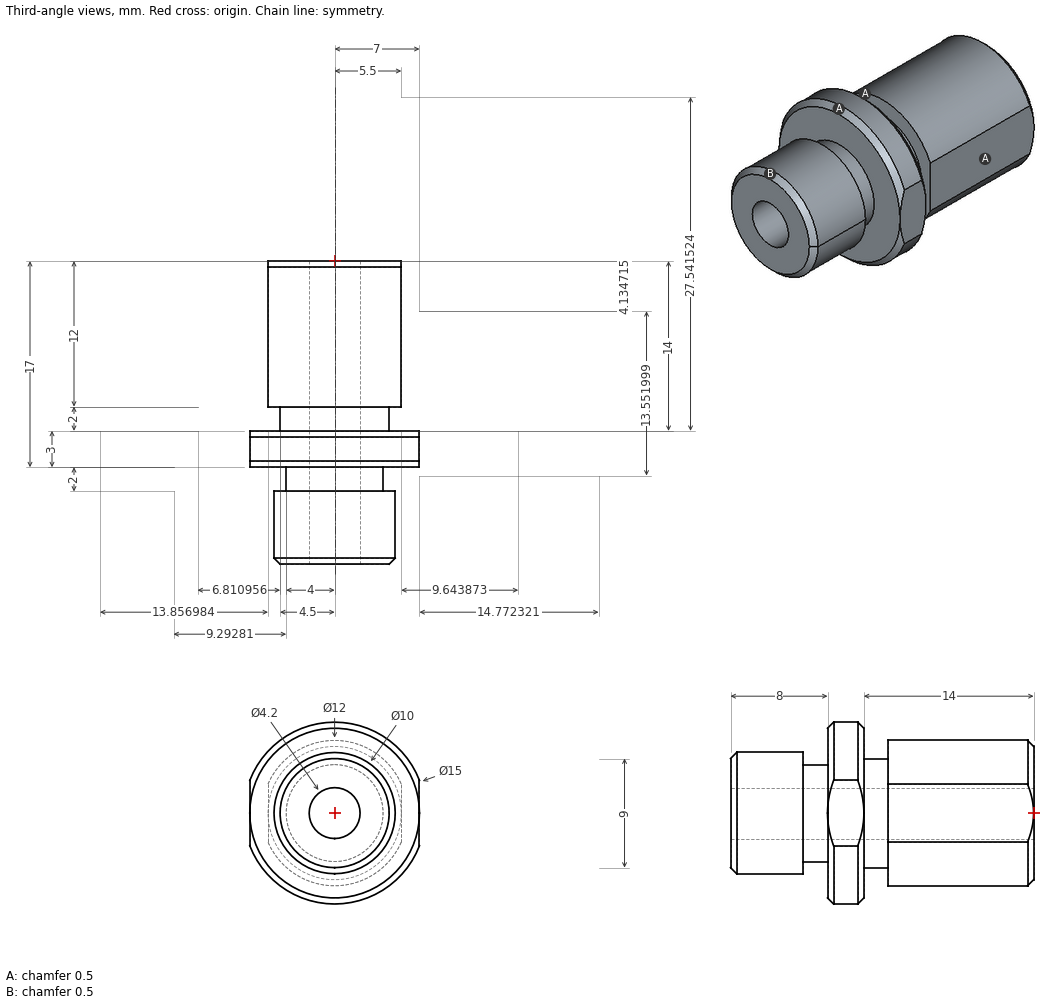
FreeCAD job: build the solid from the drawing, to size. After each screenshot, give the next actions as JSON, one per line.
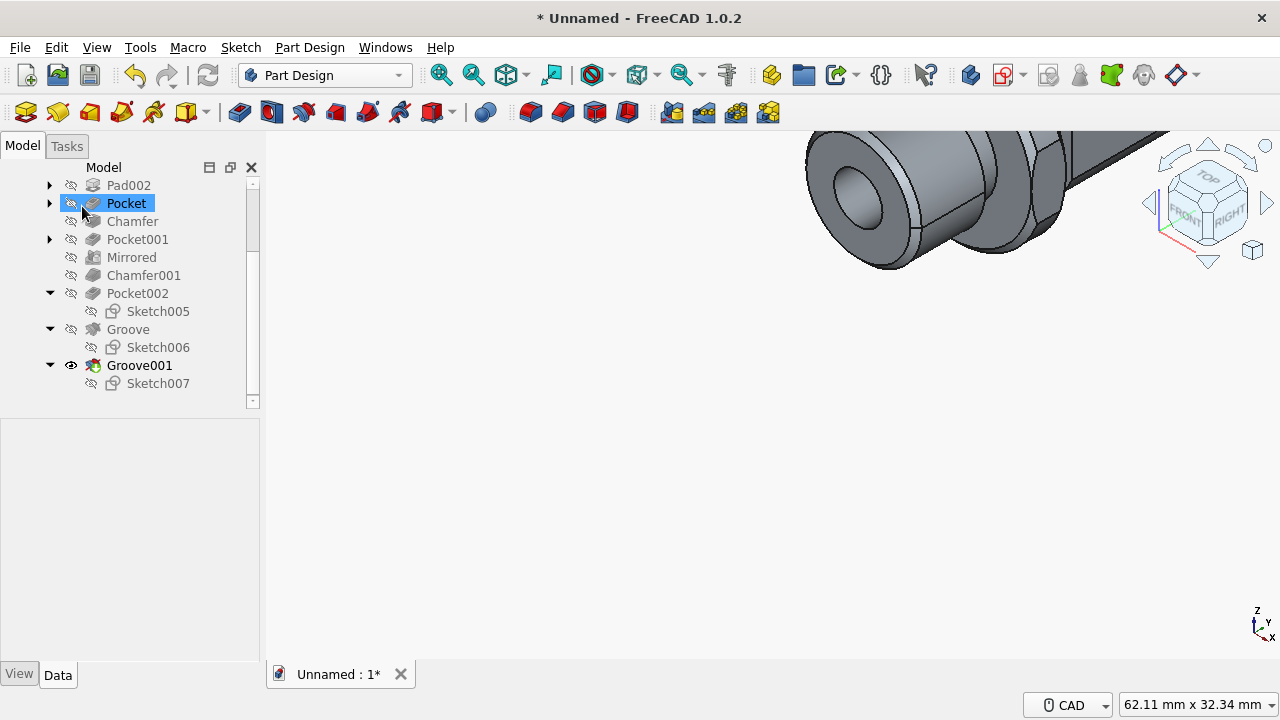
{"action": "left_click", "coordinate": [442, 76]}